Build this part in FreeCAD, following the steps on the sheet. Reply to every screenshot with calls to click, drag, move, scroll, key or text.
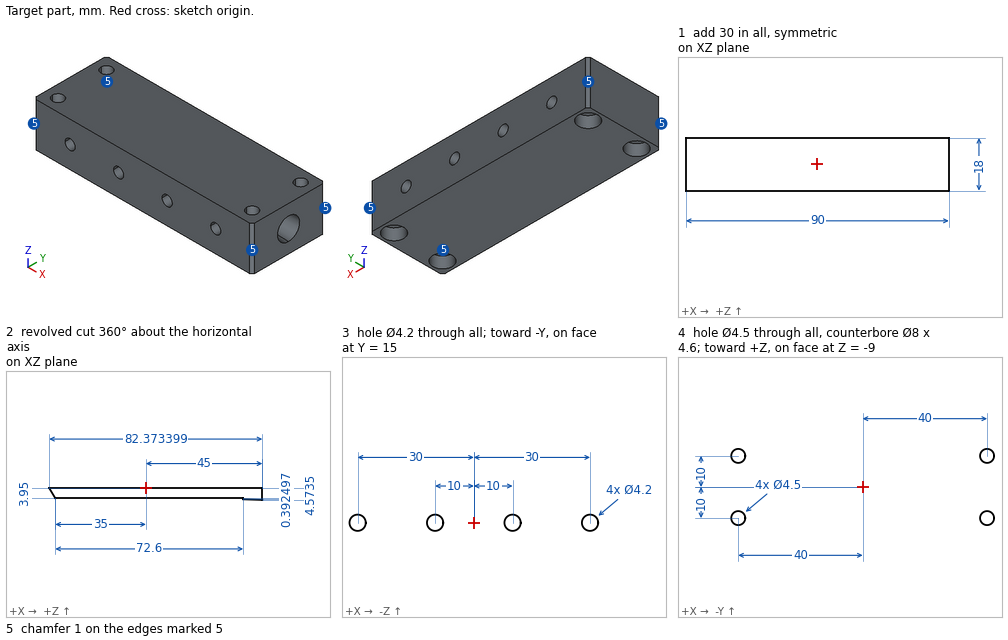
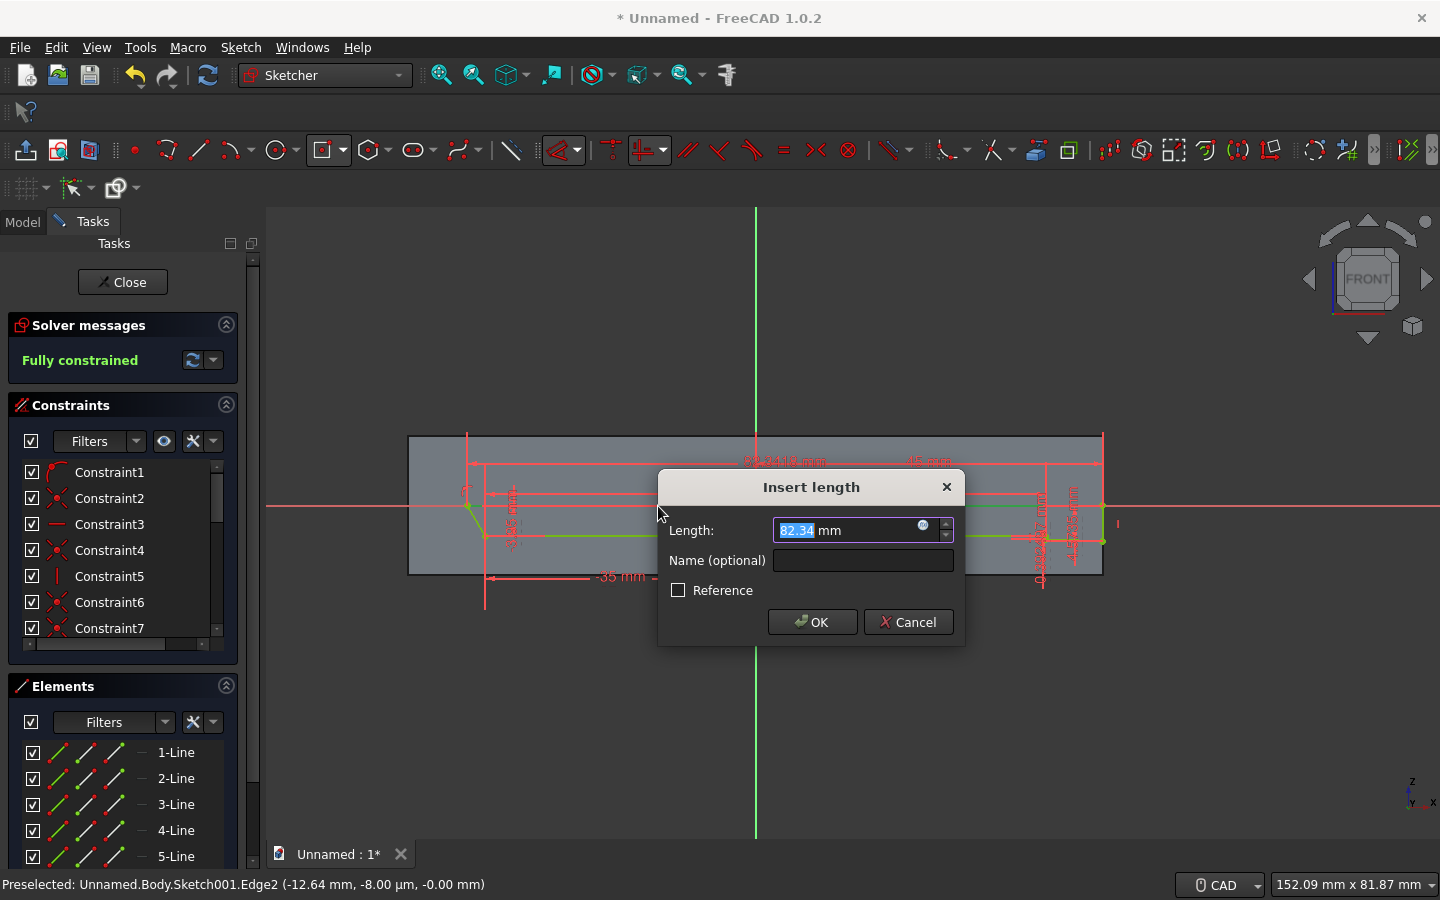
text(82.373399)
key(Return)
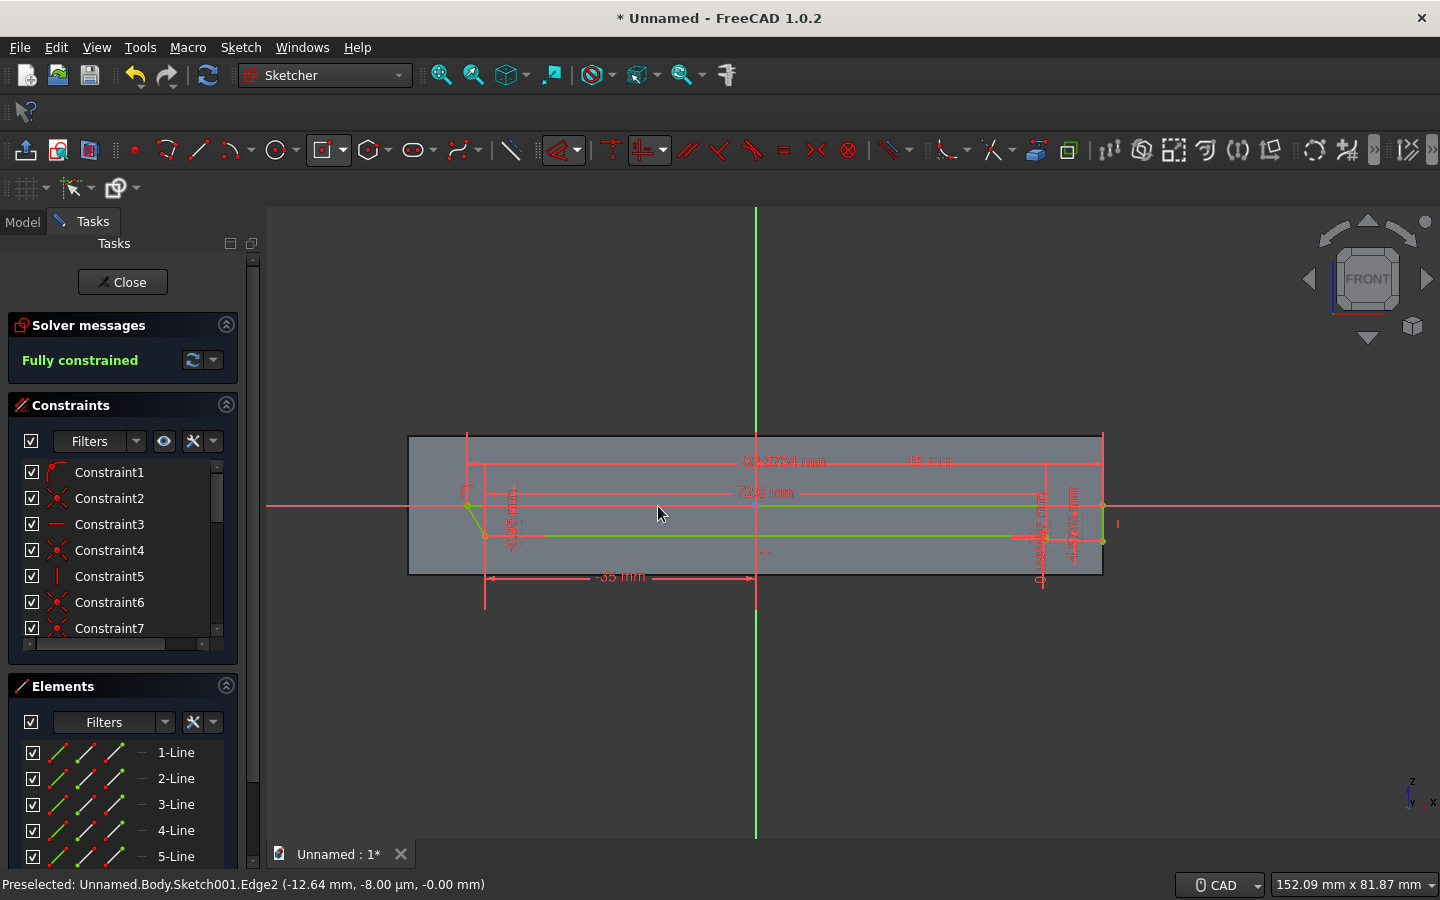
click(123, 282)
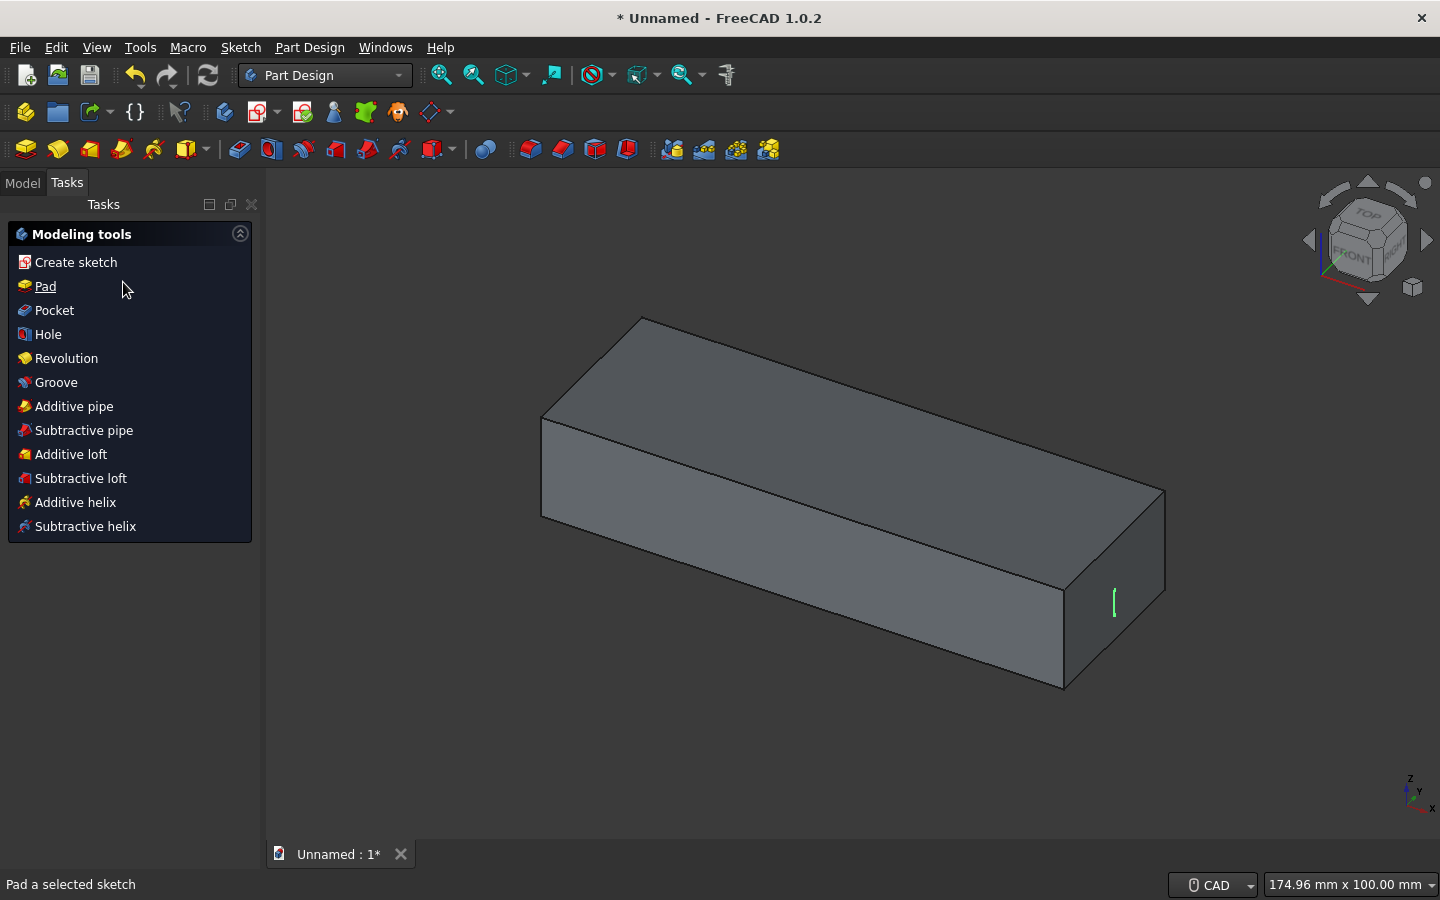
click(304, 150)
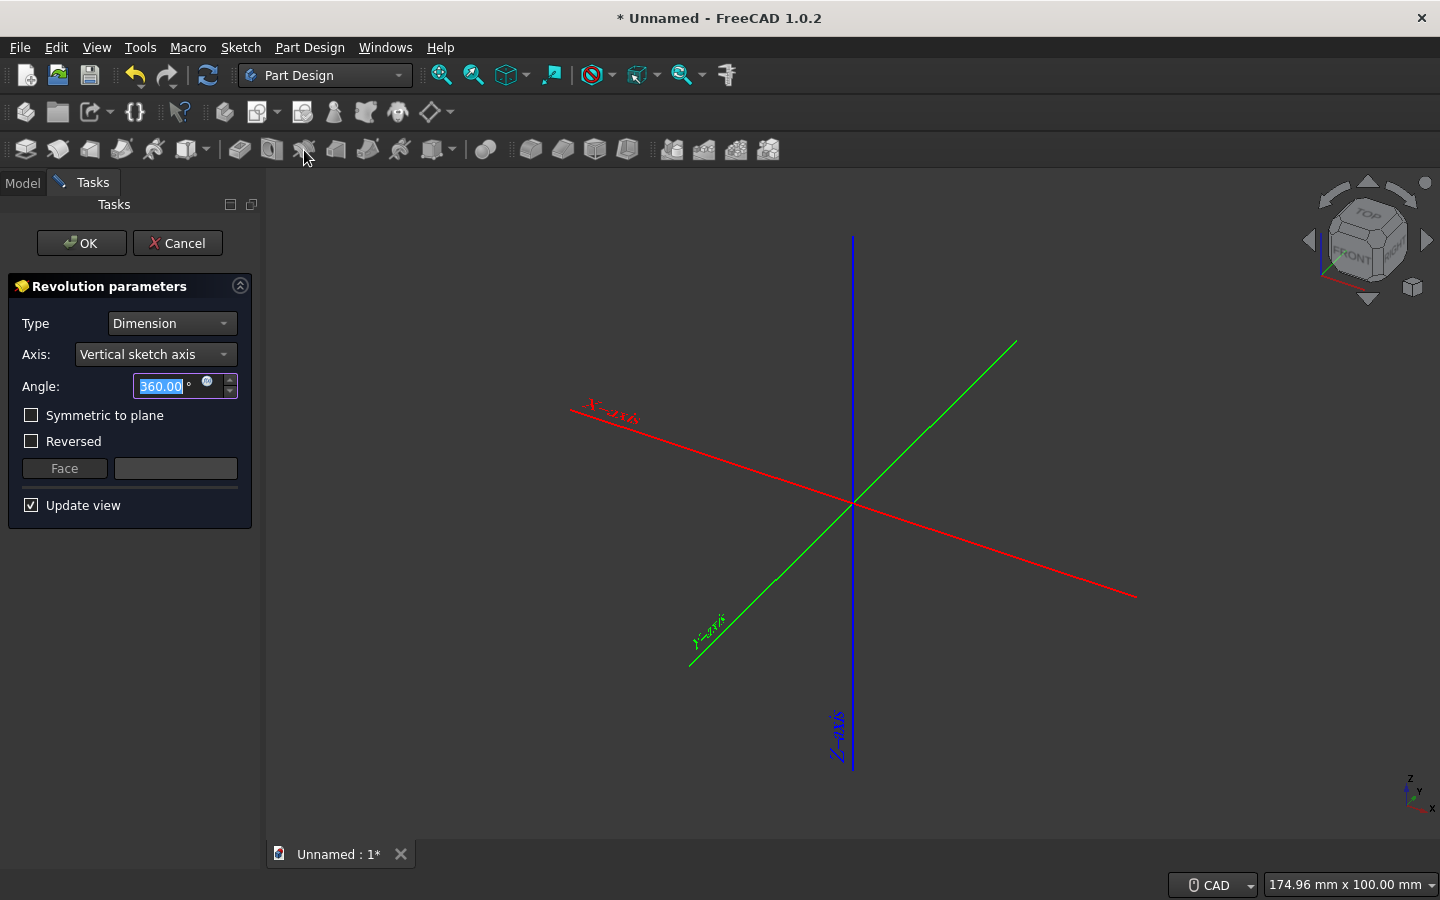
click(156, 354)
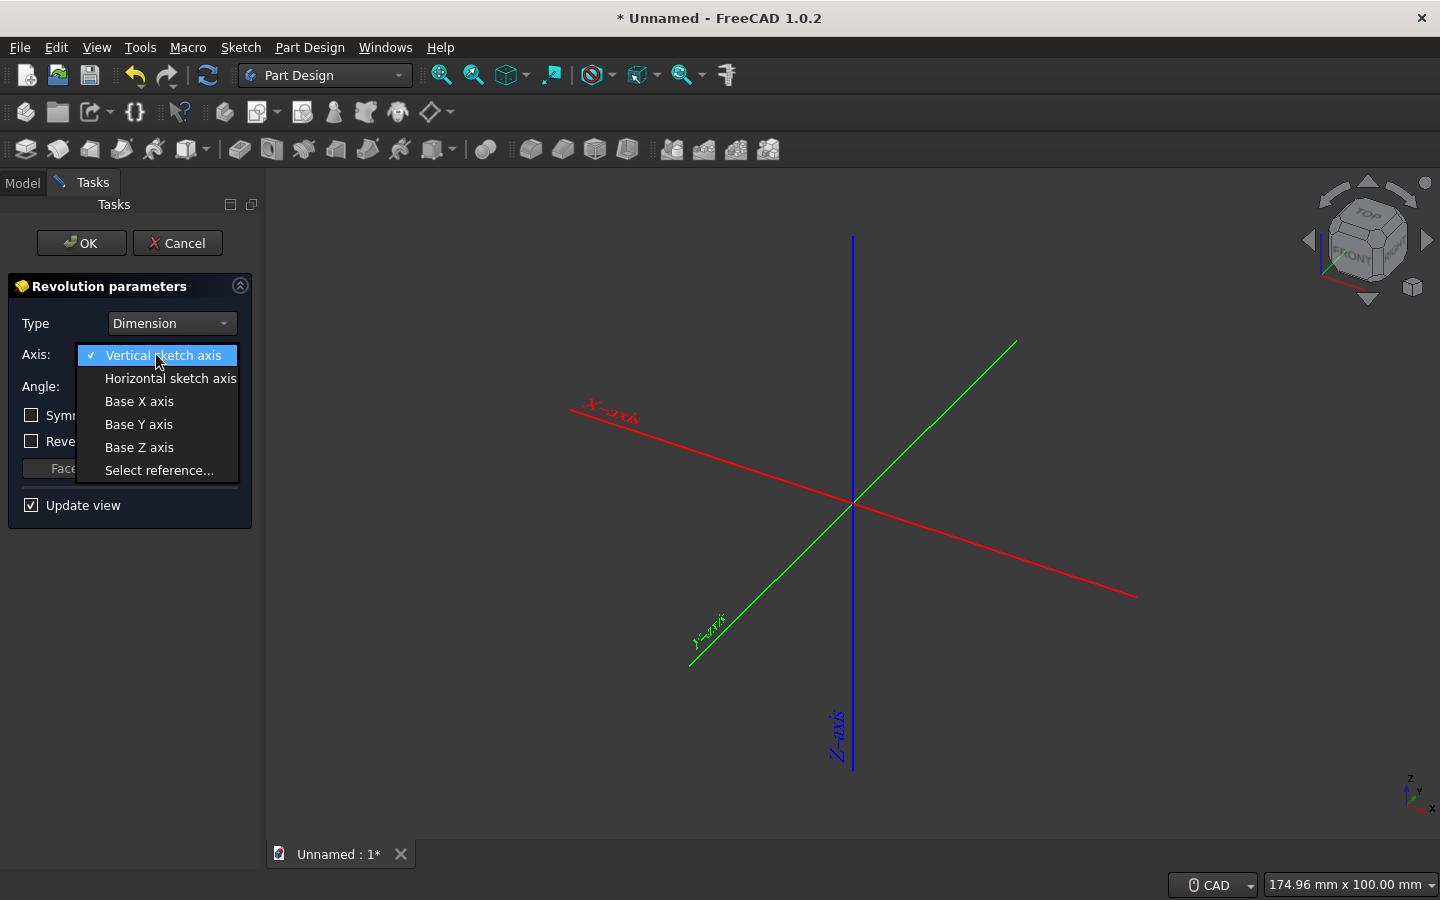
click(156, 378)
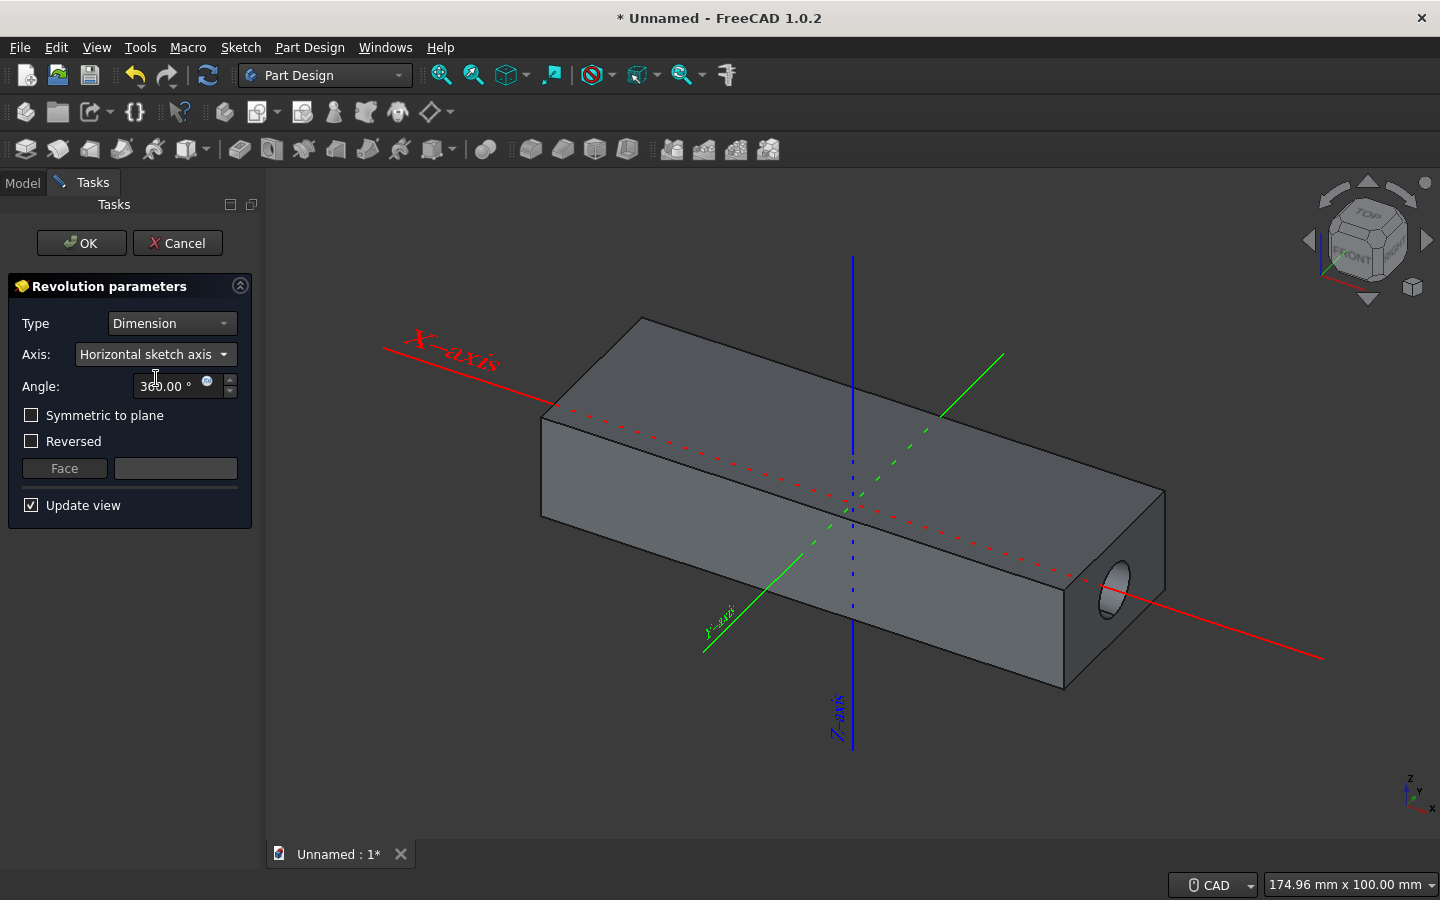
click(82, 243)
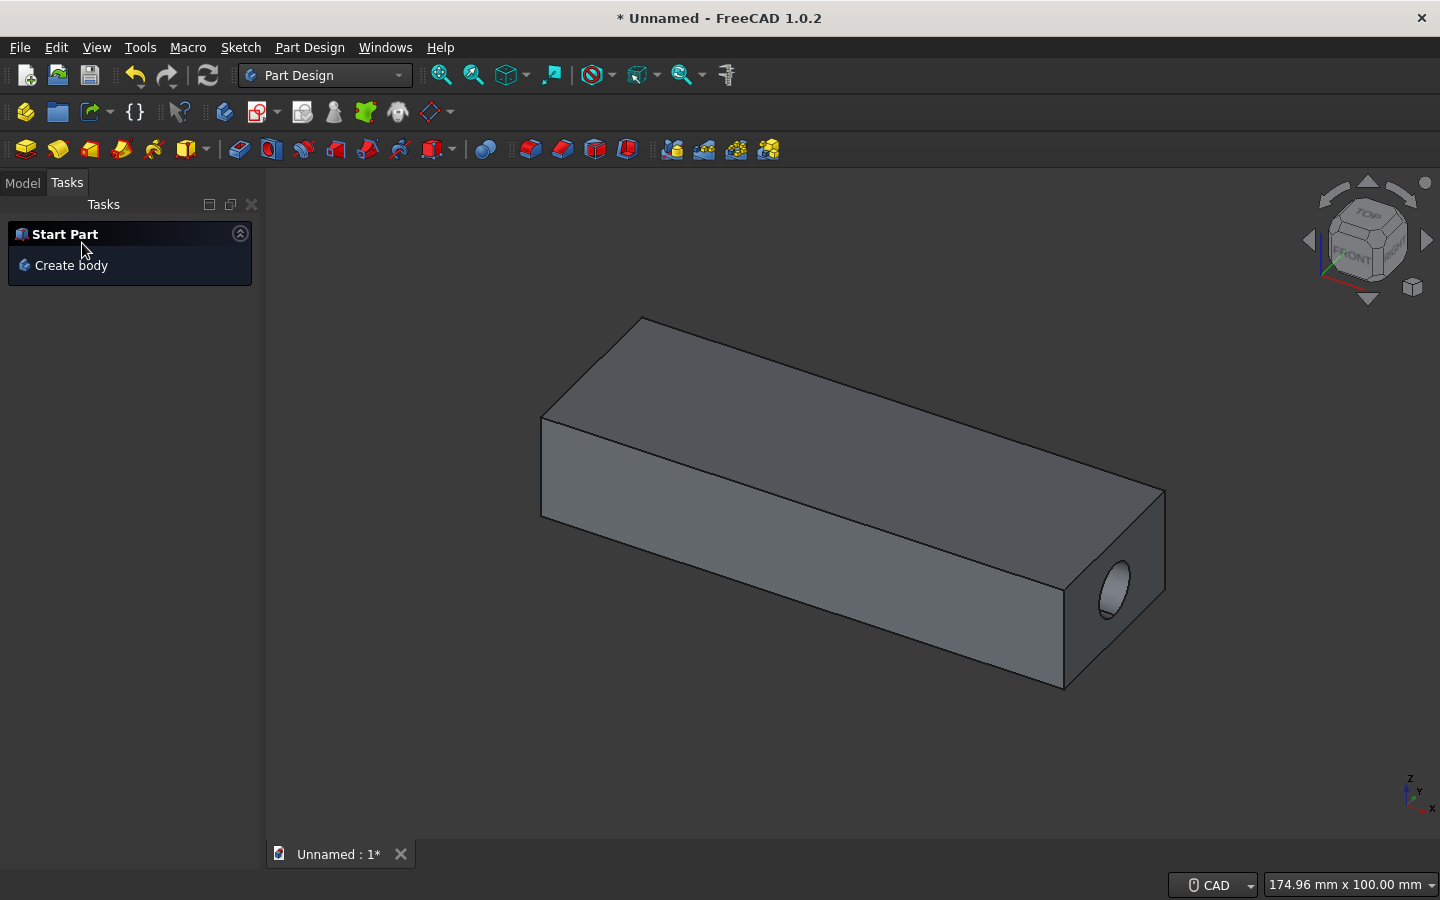
key(4)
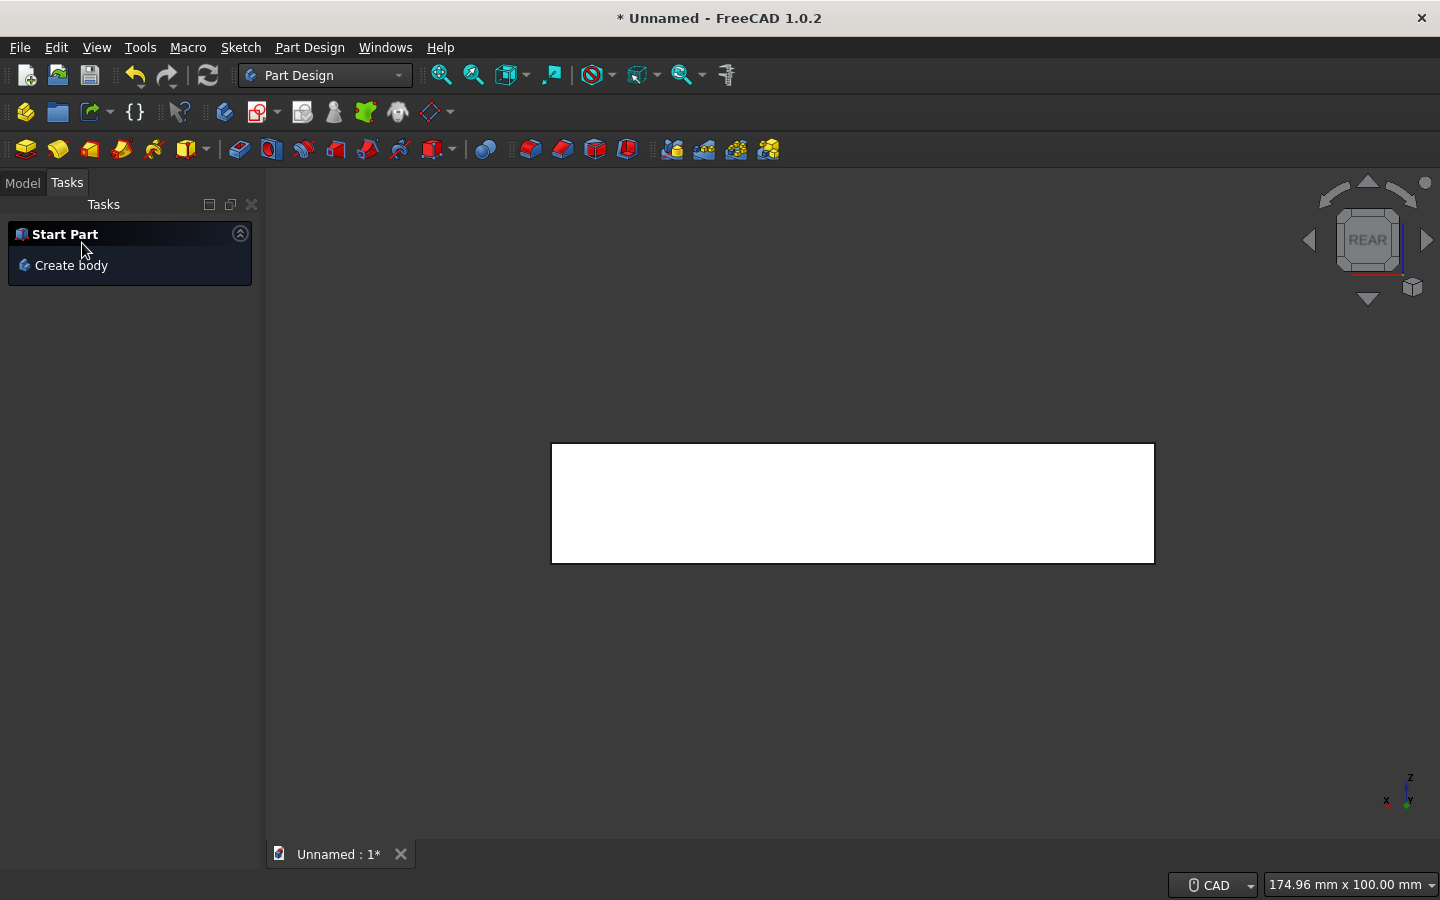
click(680, 502)